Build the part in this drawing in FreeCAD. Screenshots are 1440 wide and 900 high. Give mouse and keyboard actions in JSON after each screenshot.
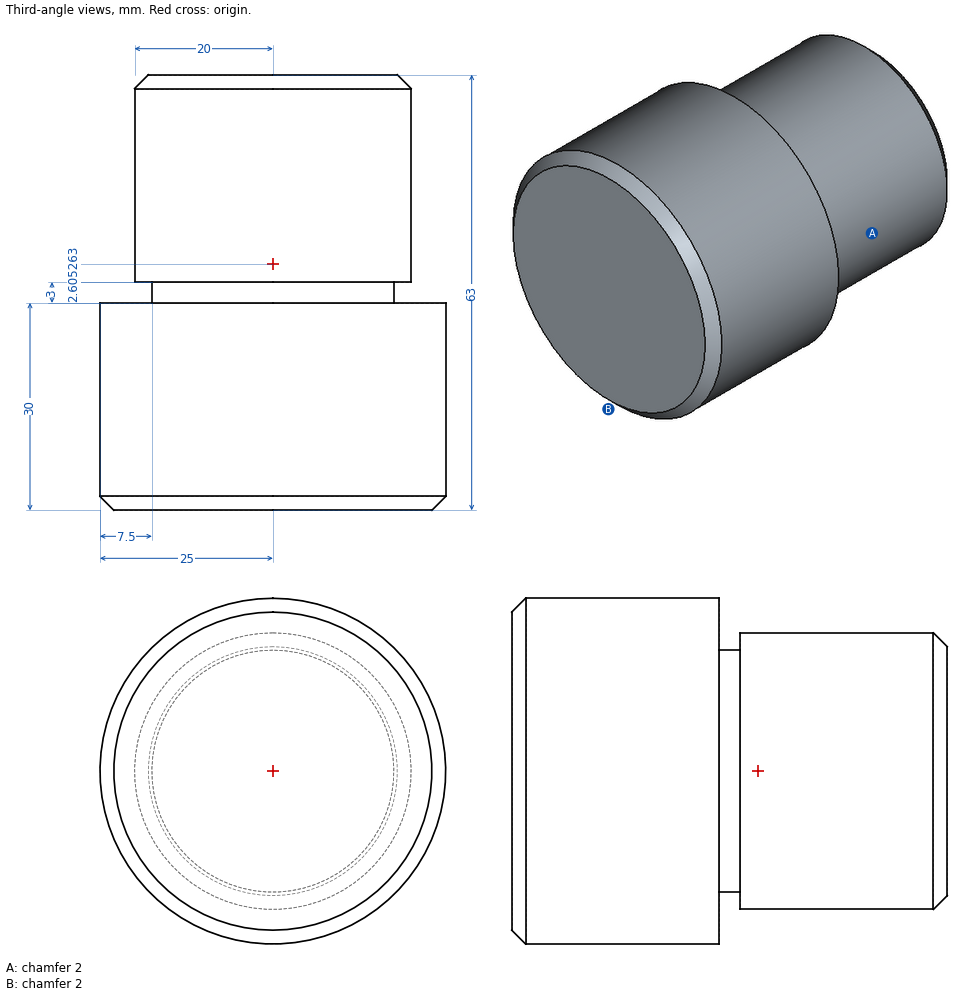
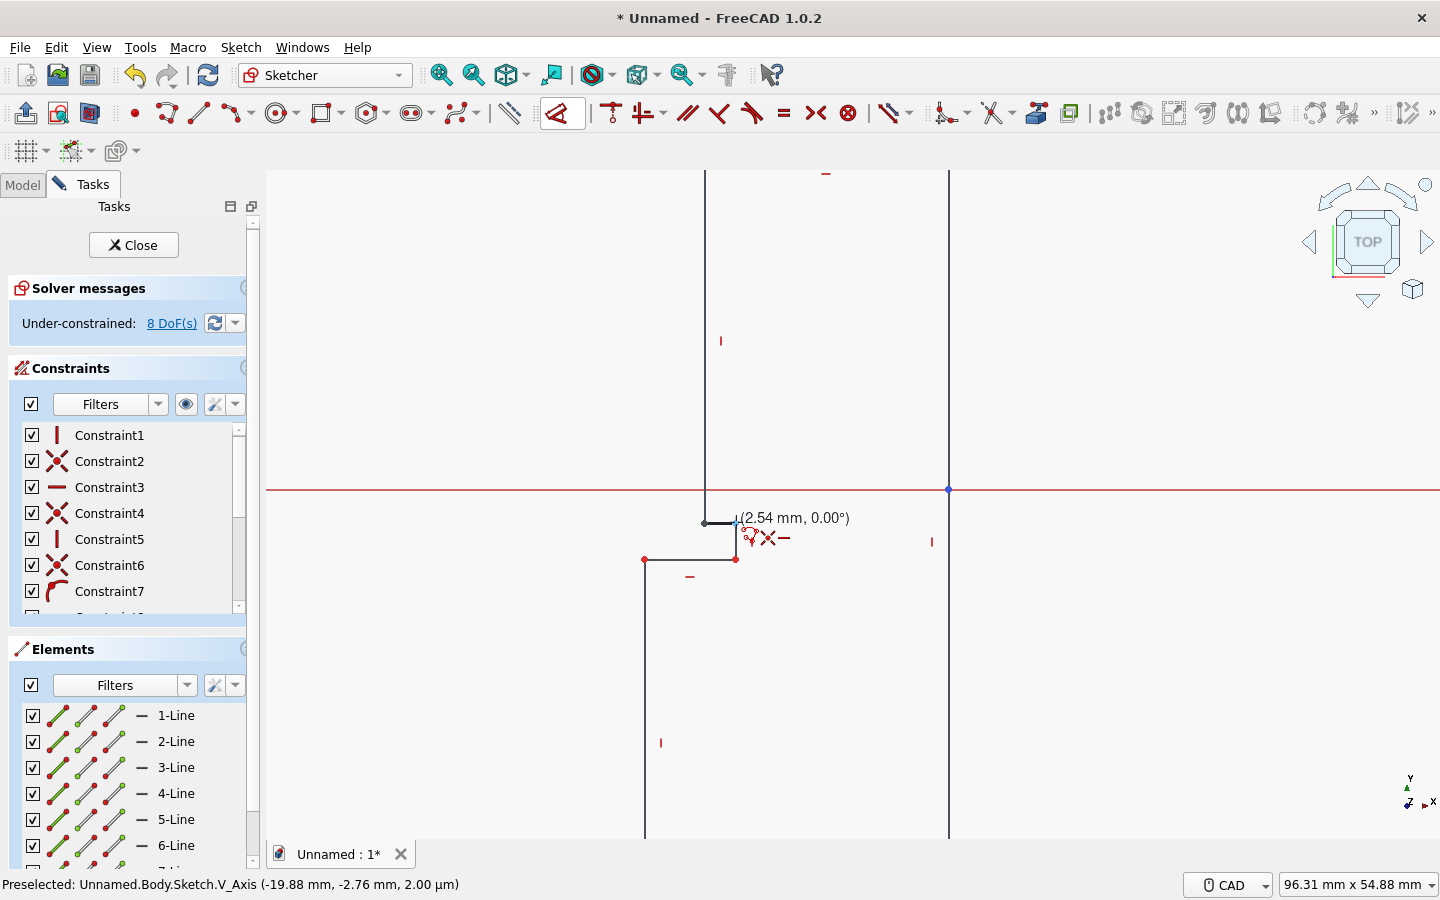
{"action": "left_click", "coordinate": [736, 523]}
{"action": "key", "text": "Escape"}
{"action": "key", "text": "Escape"}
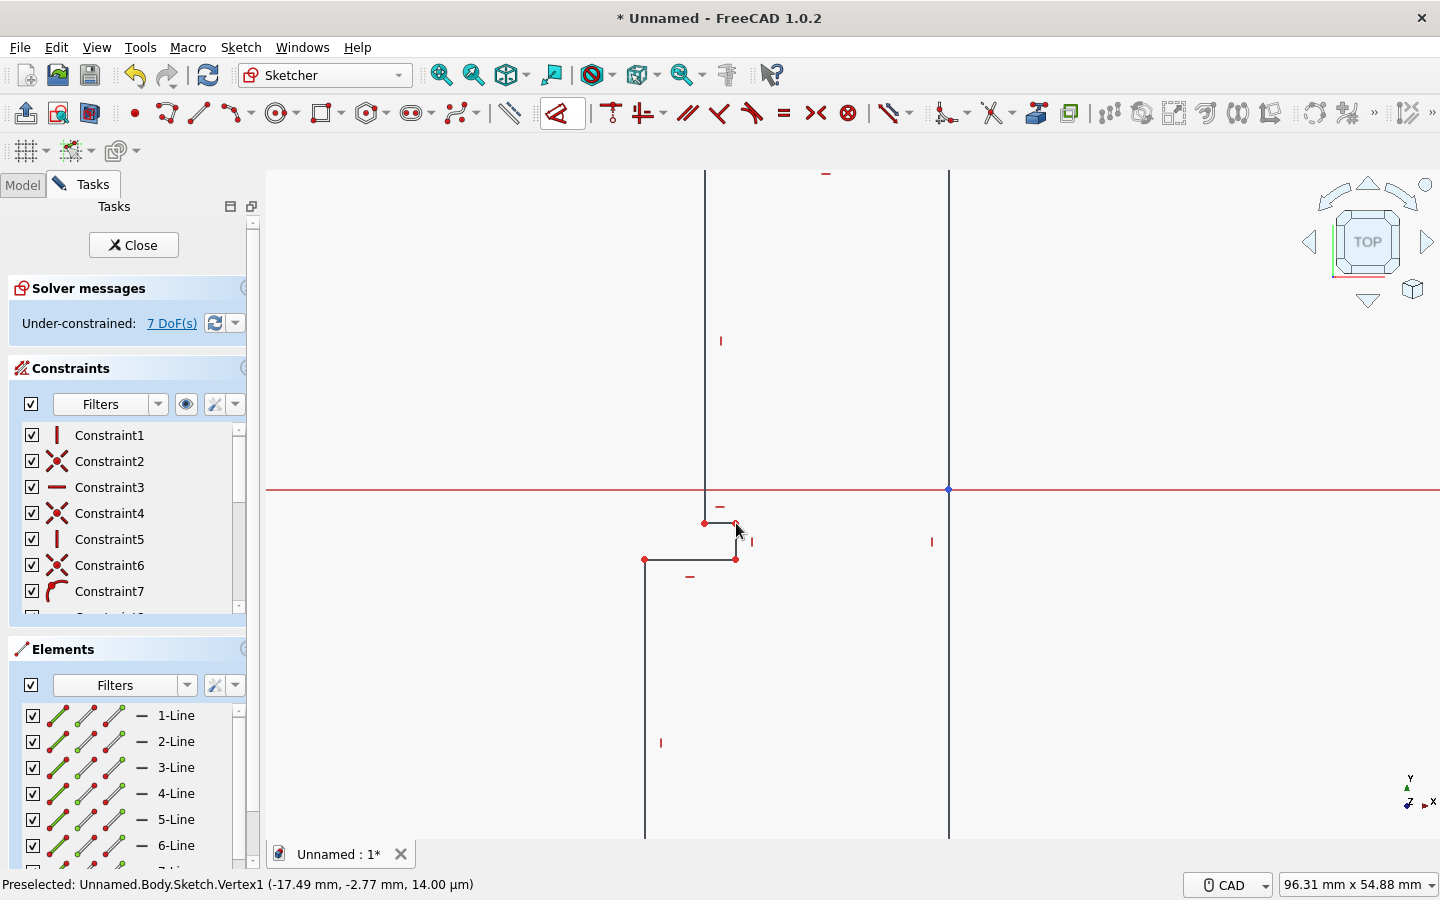
{"action": "scroll", "coordinate": [736, 534], "scroll_direction": "up", "scroll_amount": 2}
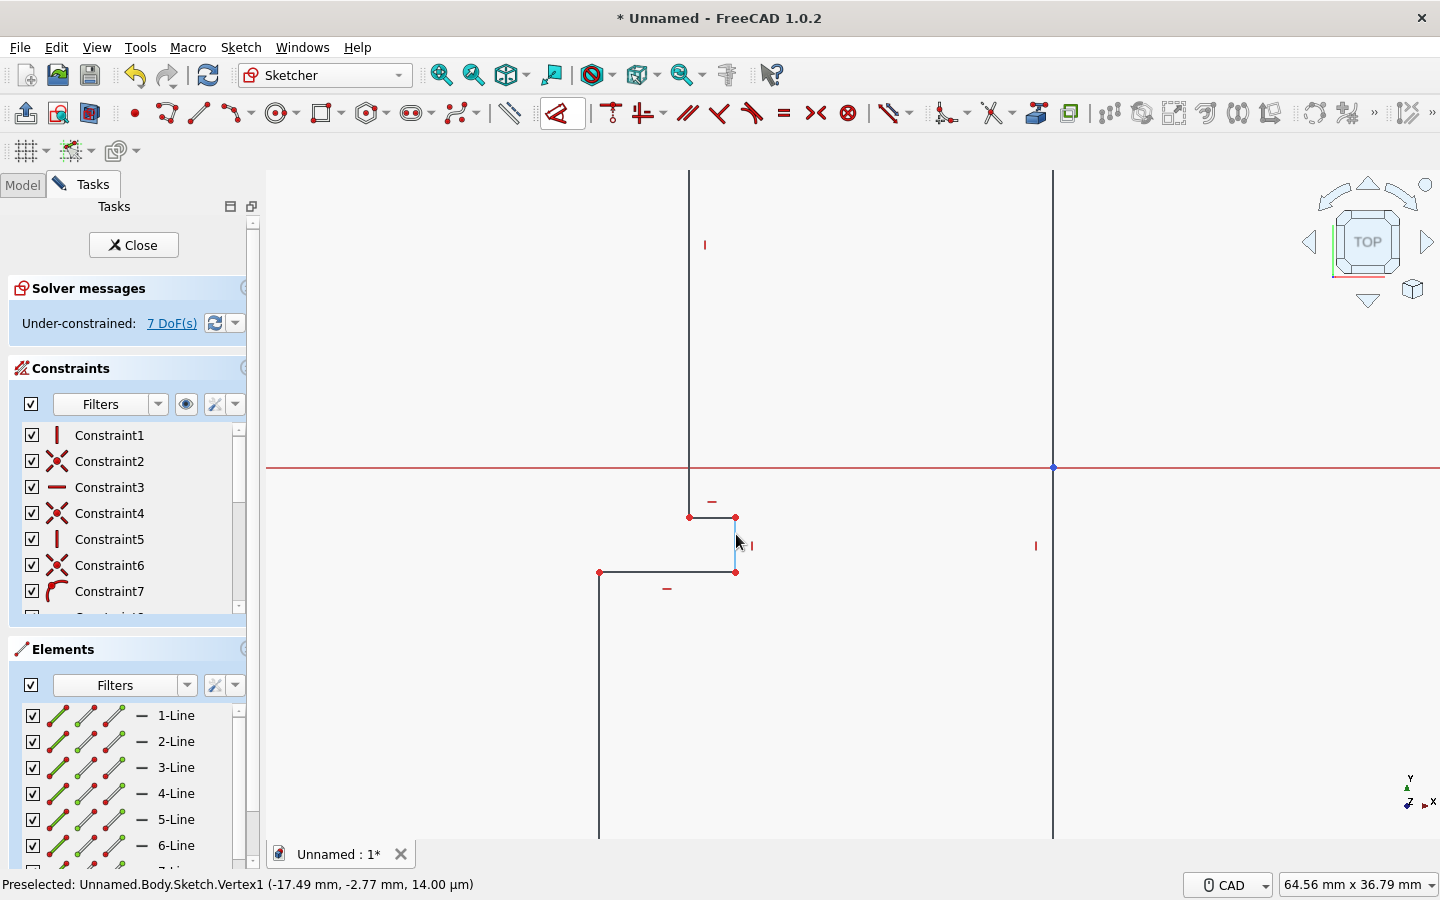
{"action": "left_click", "coordinate": [735, 534]}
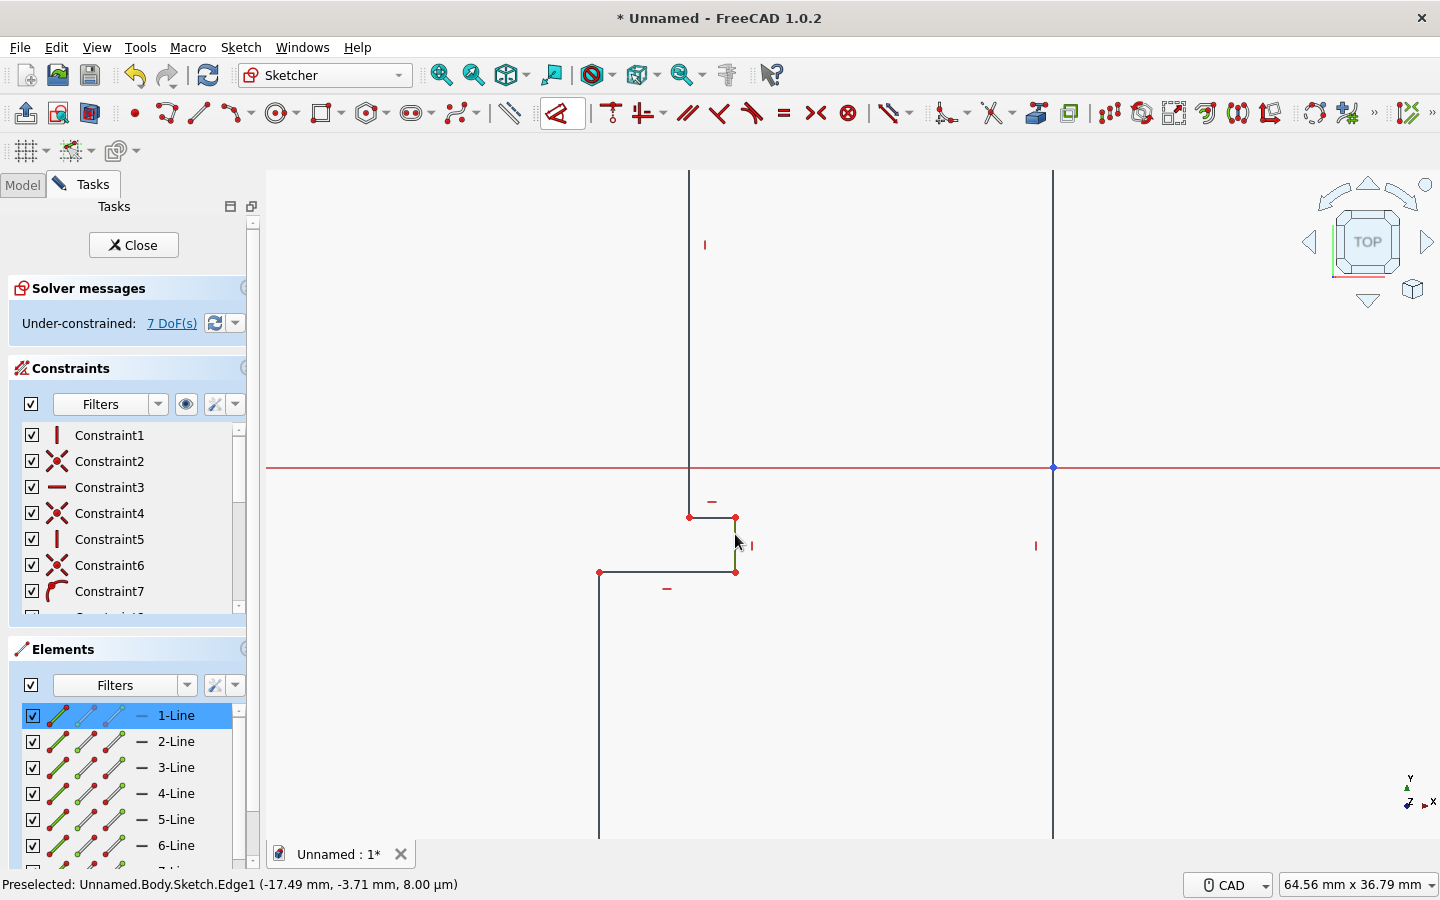
{"action": "key", "text": "i"}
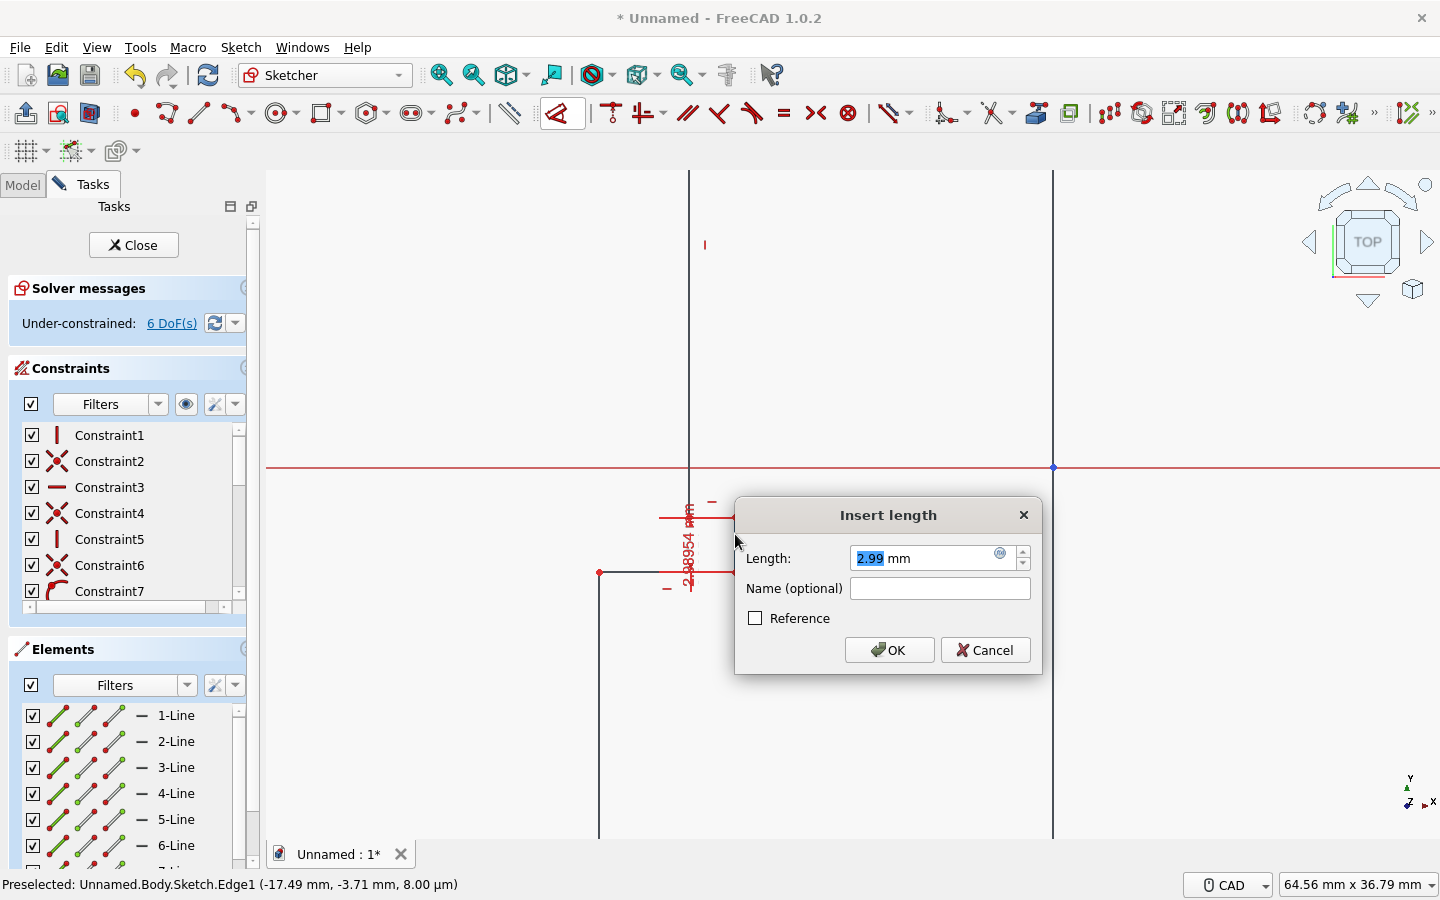
{"action": "type", "text": "3"}
{"action": "key", "text": "Return"}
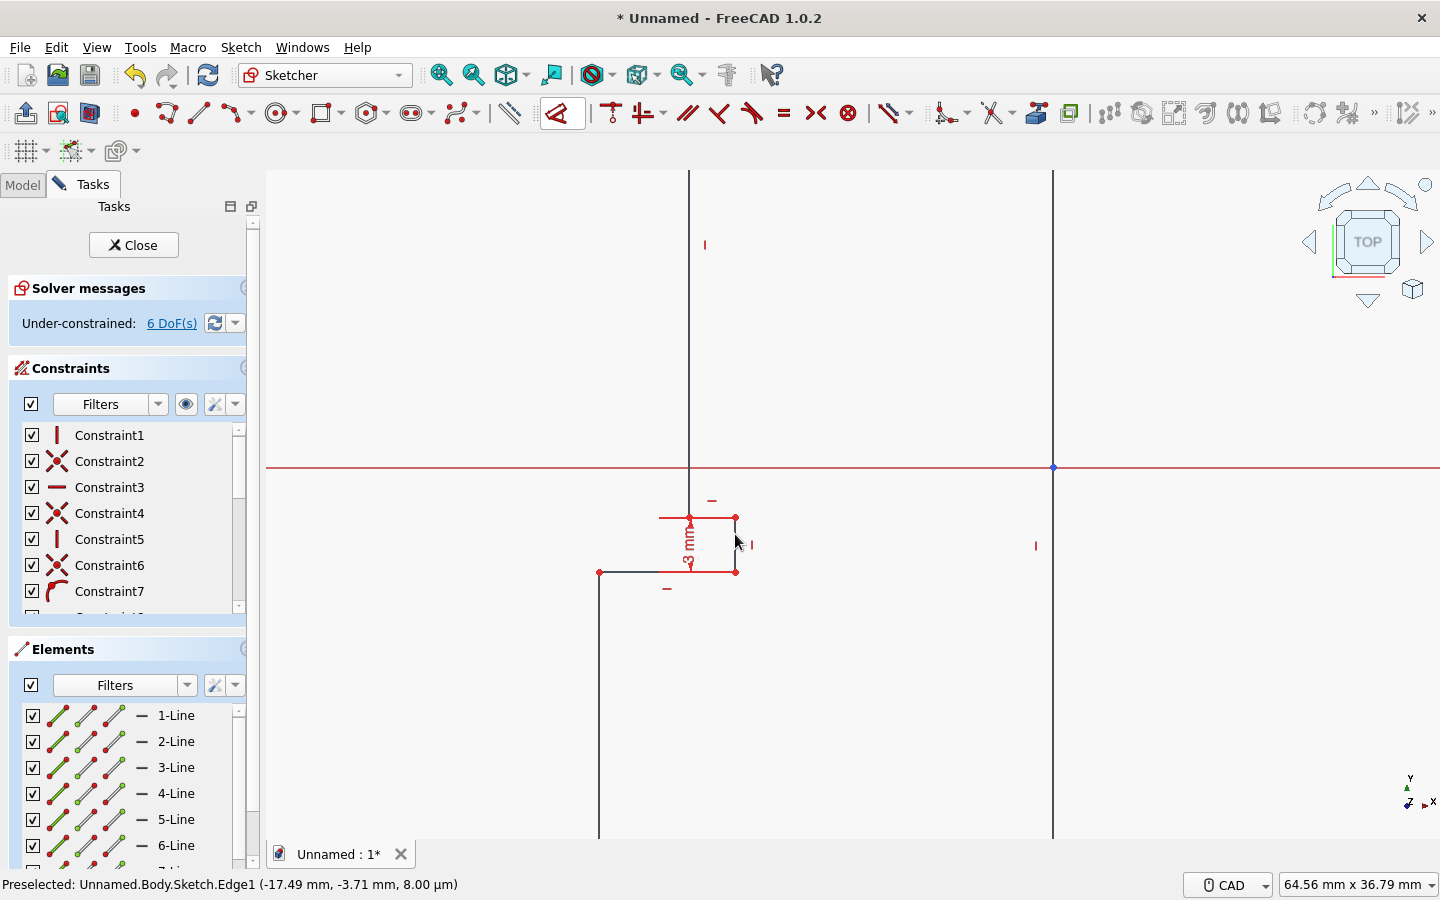
{"action": "left_click", "coordinate": [599, 736]}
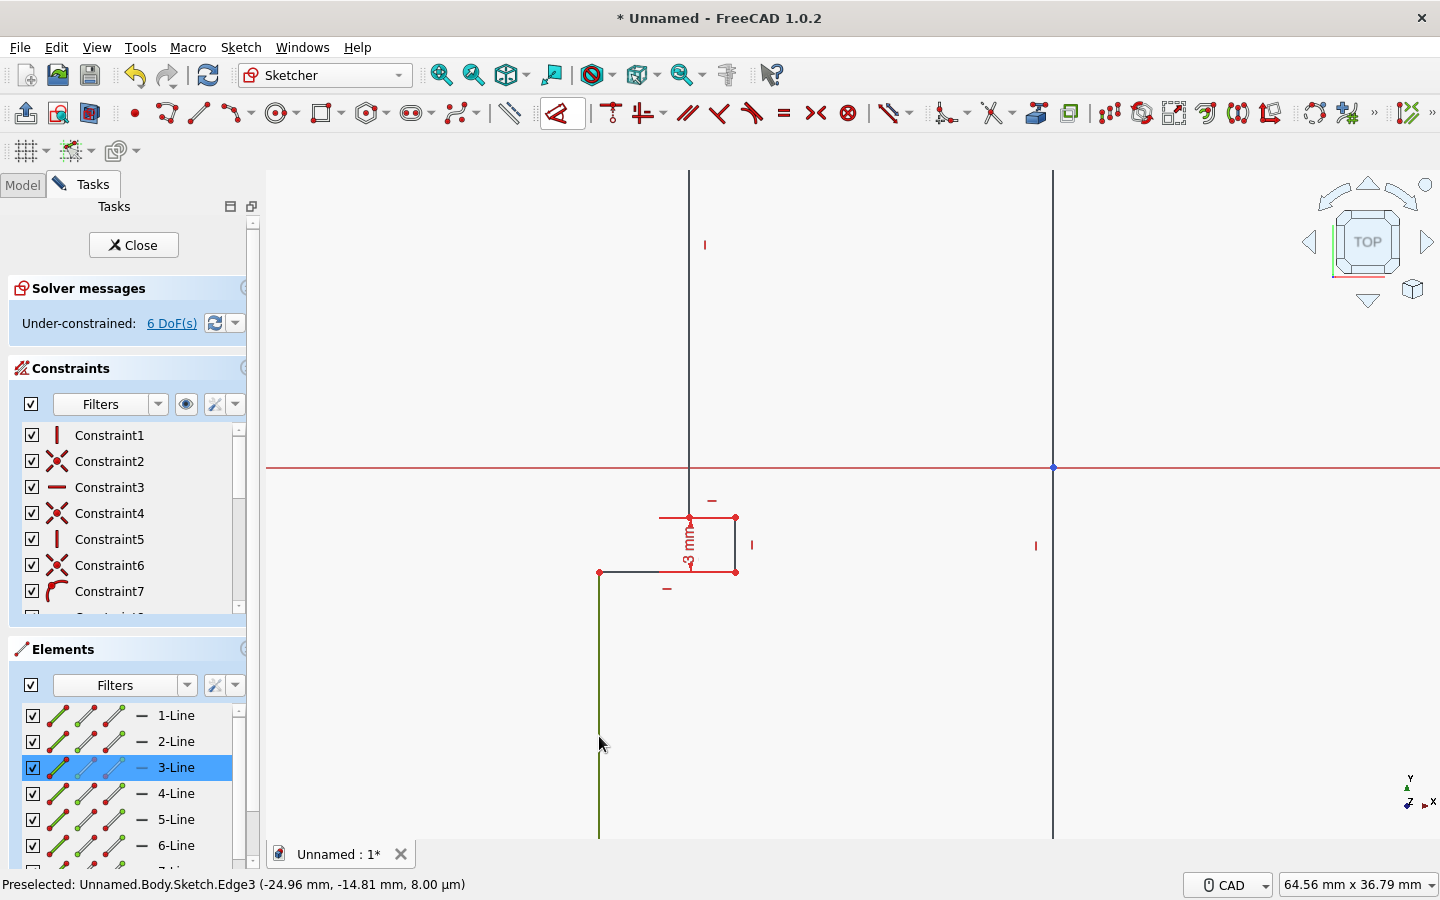
{"action": "left_click", "coordinate": [580, 114]}